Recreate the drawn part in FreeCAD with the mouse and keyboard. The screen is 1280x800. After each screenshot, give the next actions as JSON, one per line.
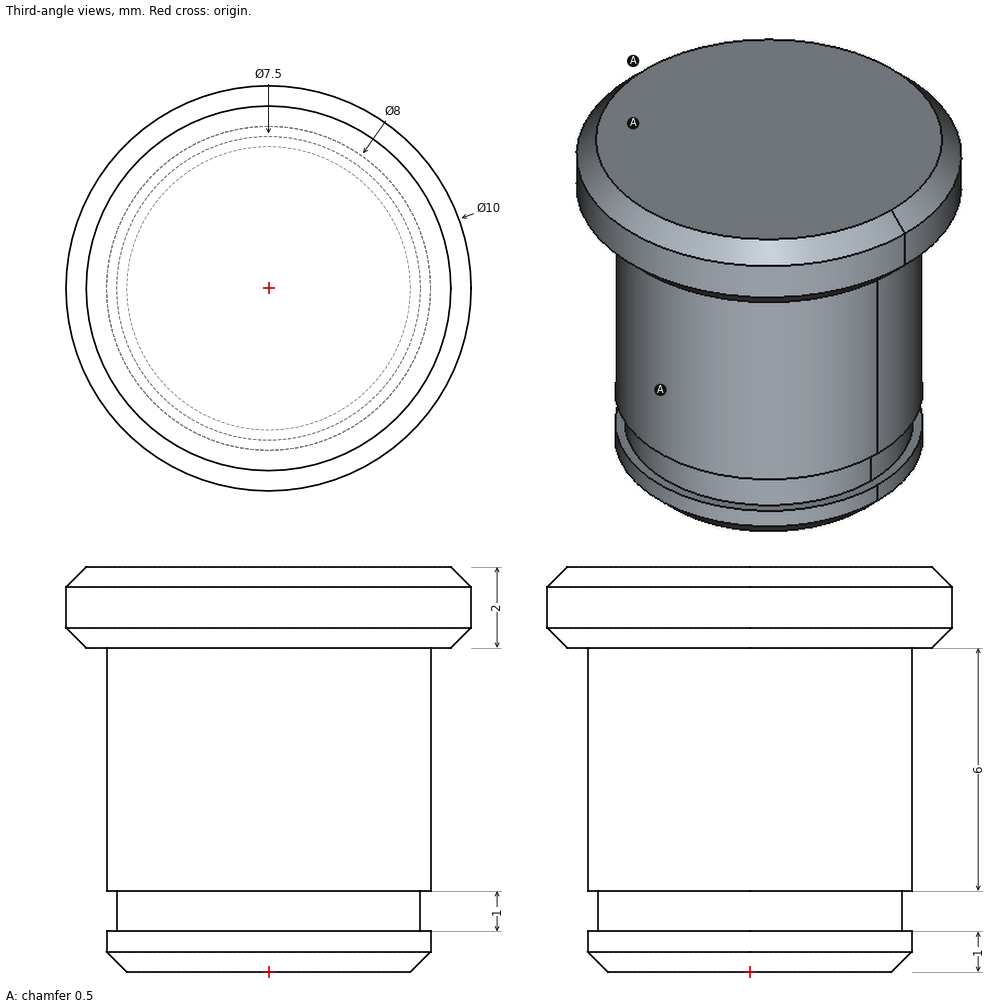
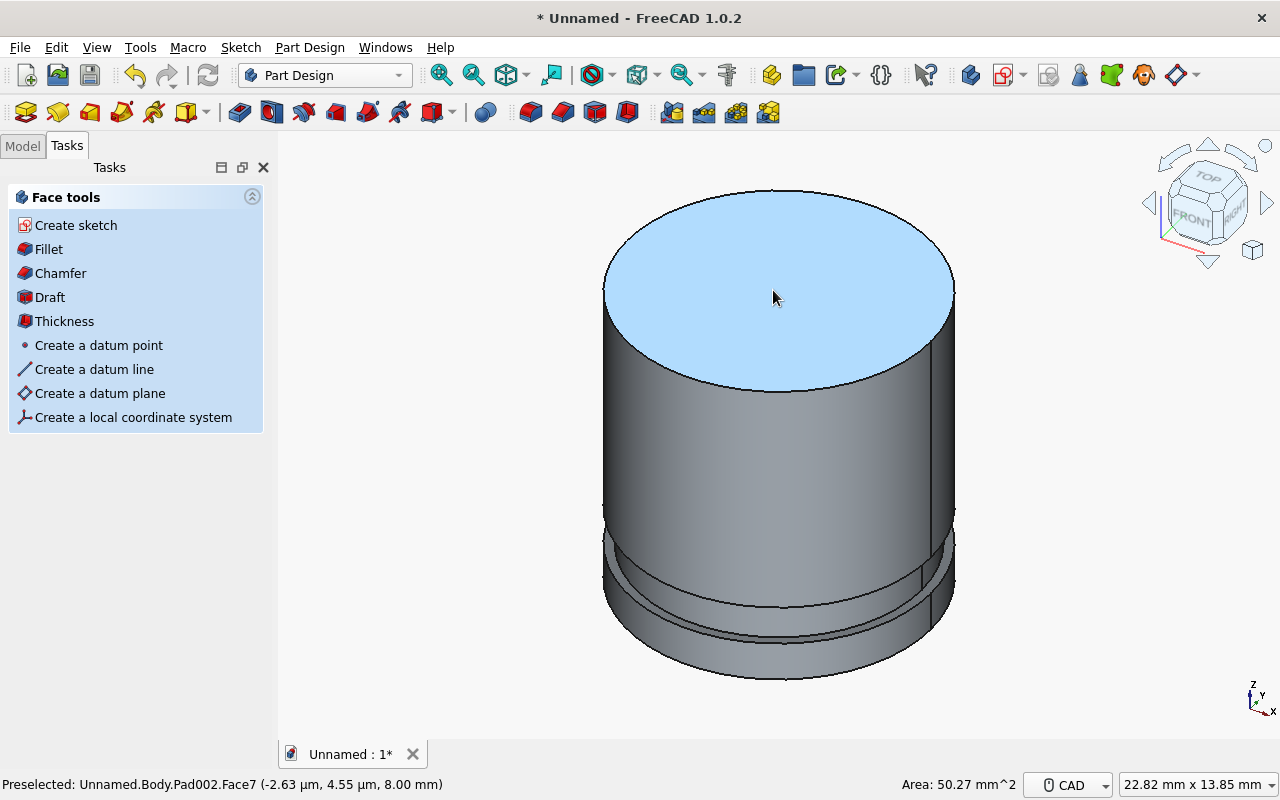
{"action": "left_click", "coordinate": [1004, 76]}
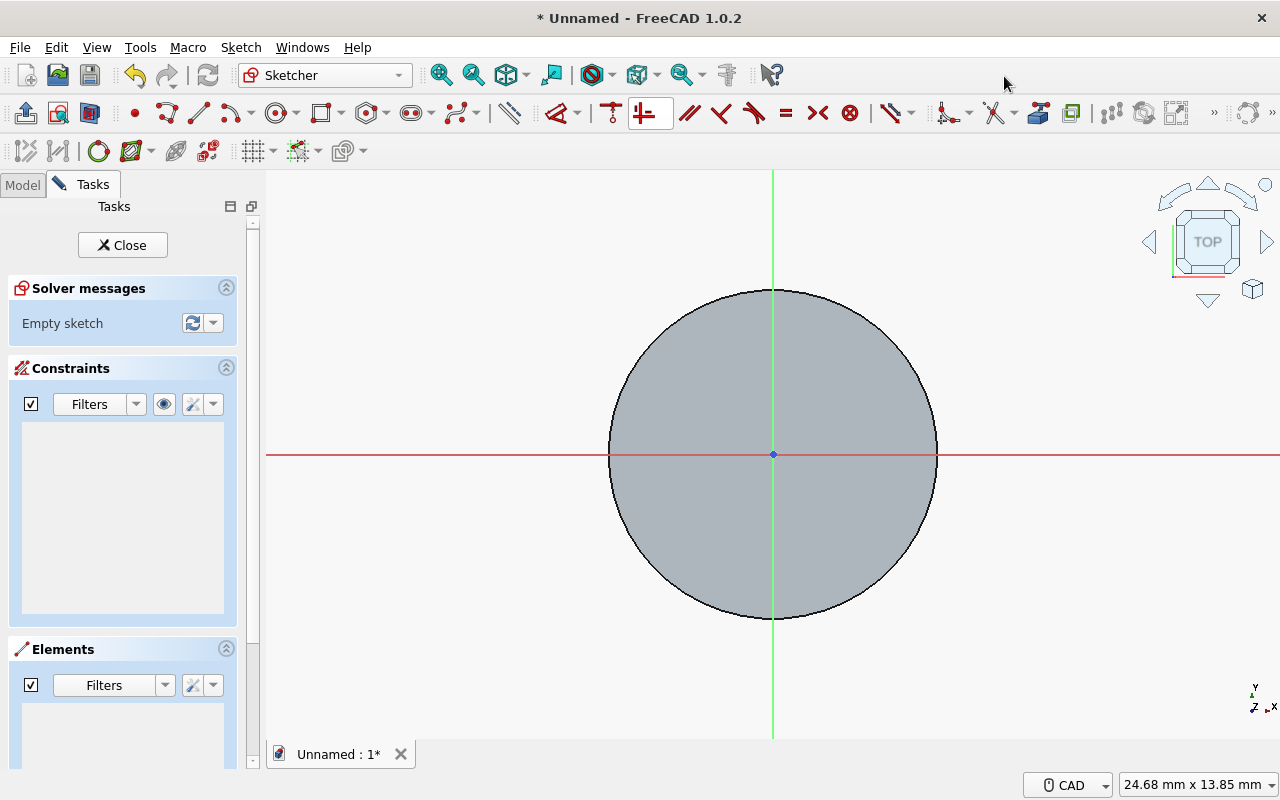
{"action": "key", "text": "g c"}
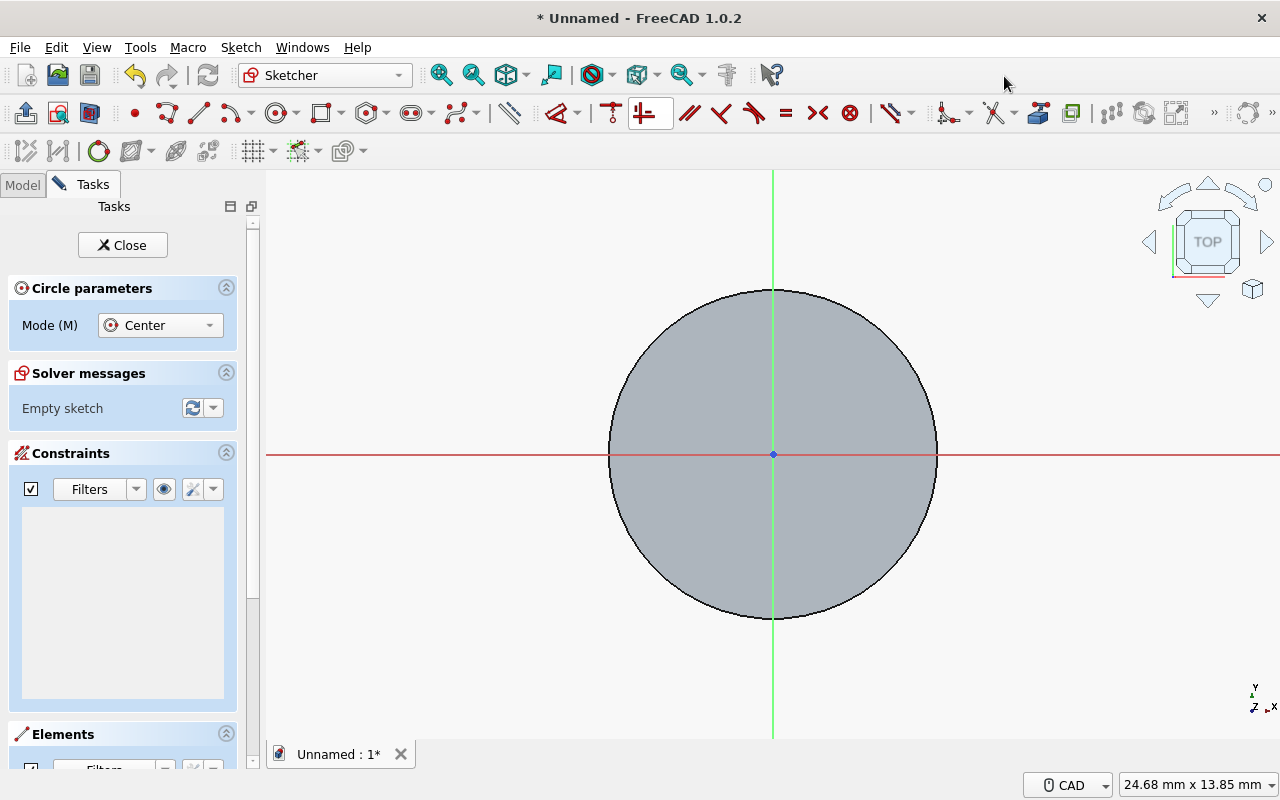
{"action": "left_click", "coordinate": [773, 454]}
{"action": "left_click", "coordinate": [918, 309]}
{"action": "key", "text": "Escape"}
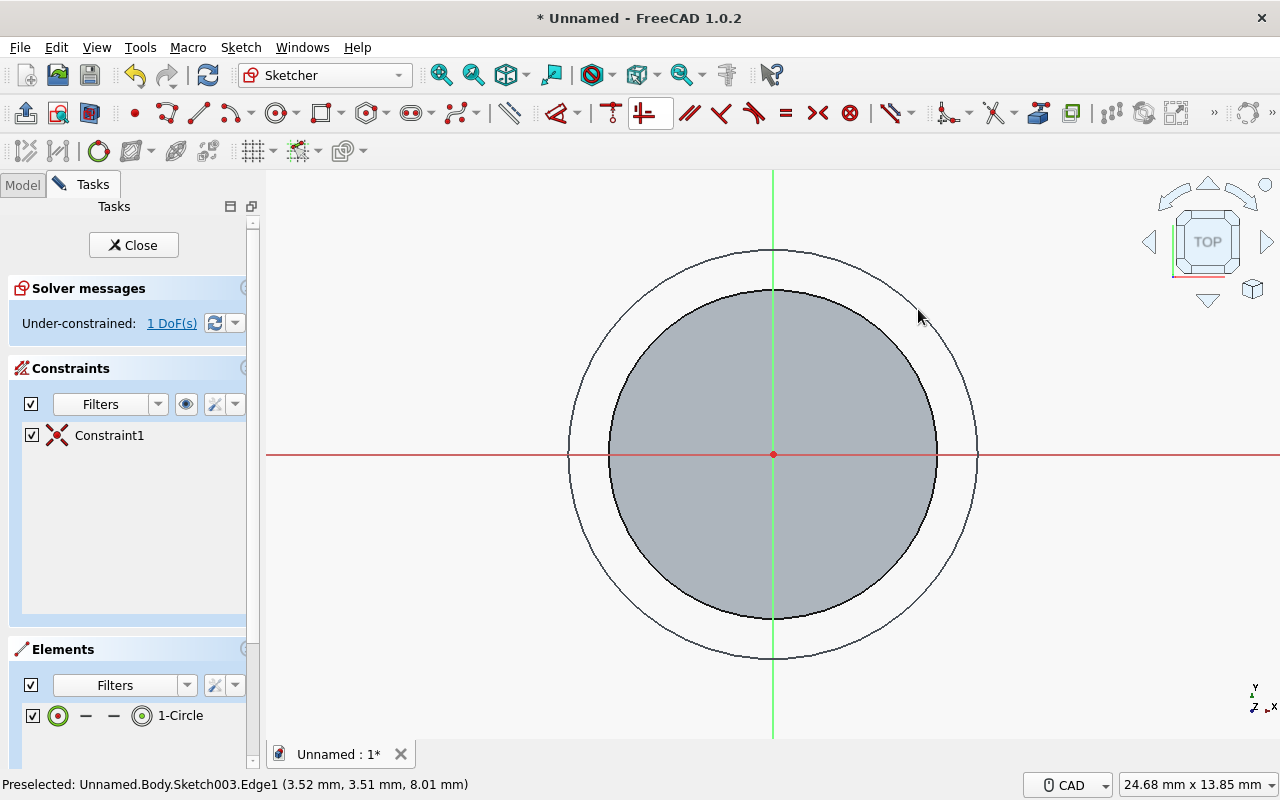
{"action": "key", "text": "d"}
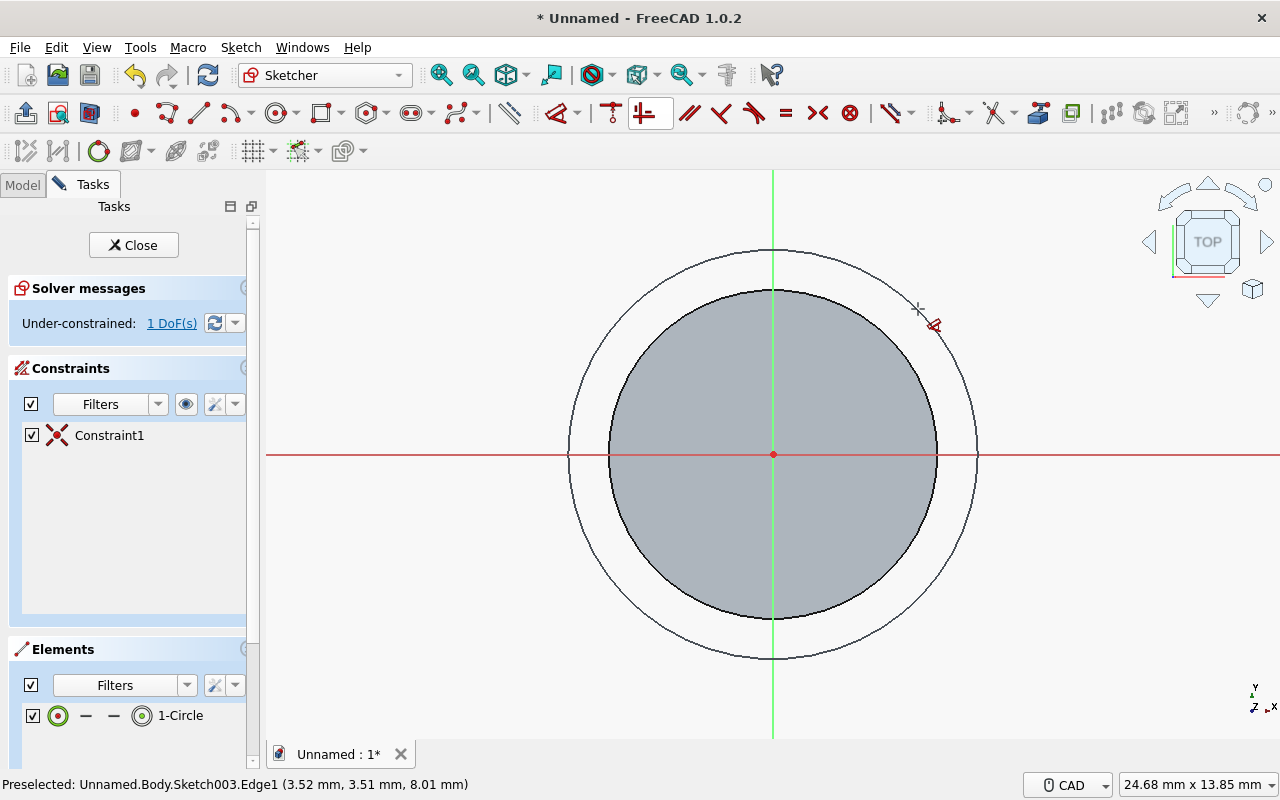
{"action": "left_click", "coordinate": [917, 309]}
{"action": "left_click", "coordinate": [940, 286]}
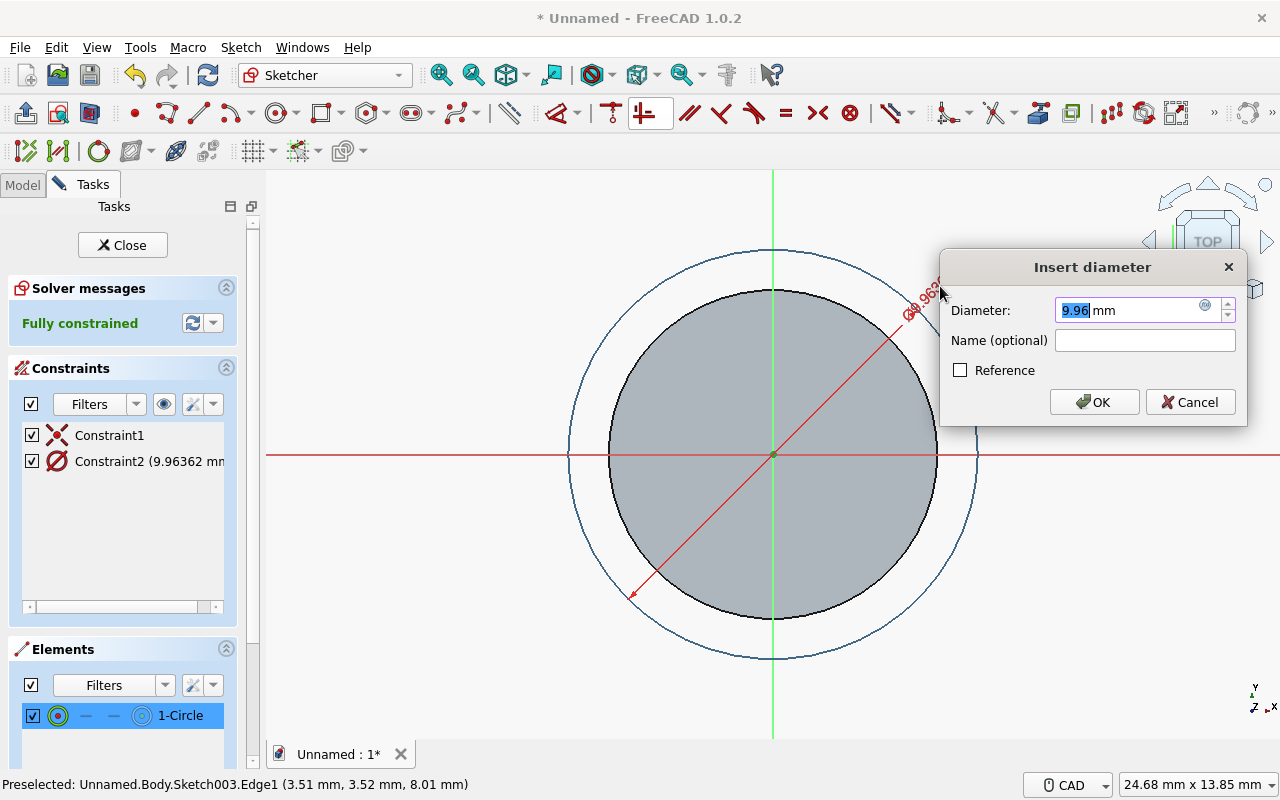
{"action": "type", "text": "10"}
{"action": "key", "text": "Return"}
{"action": "key", "text": "Escape"}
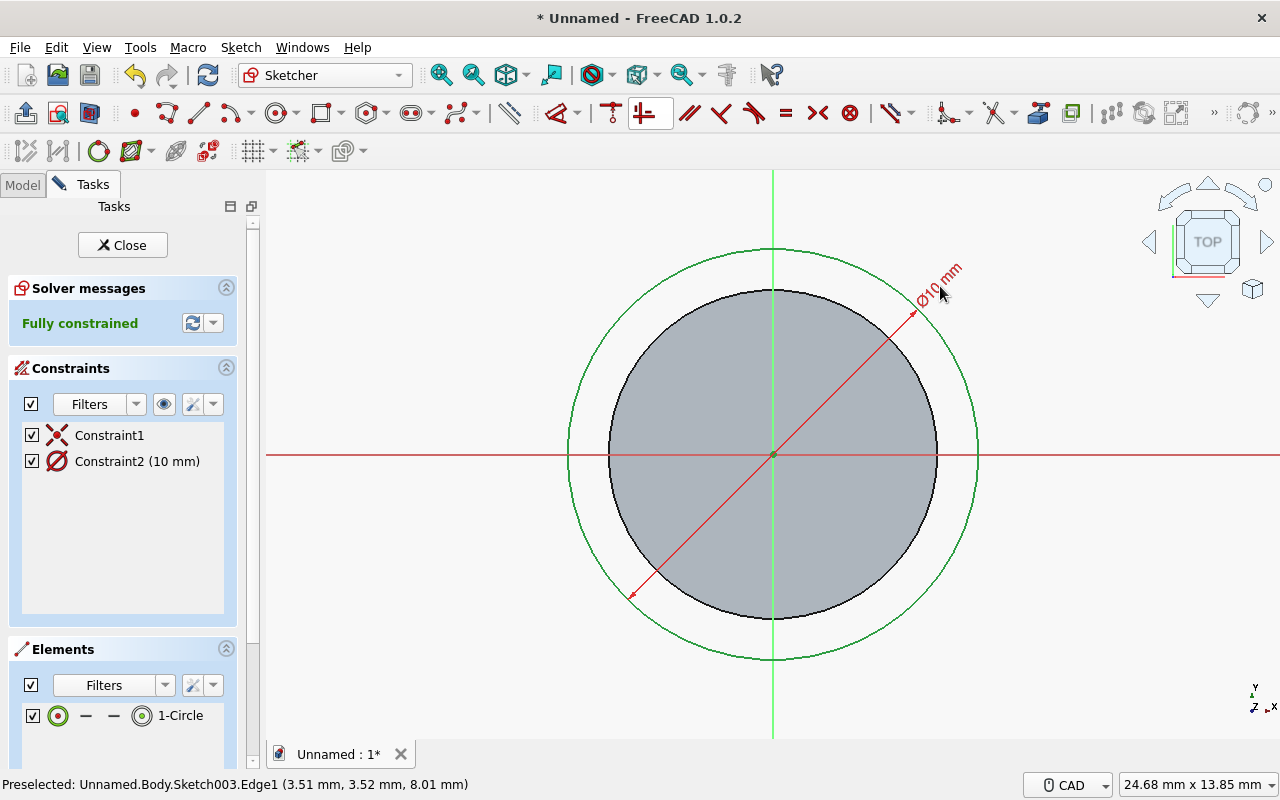
{"action": "left_click", "coordinate": [123, 245]}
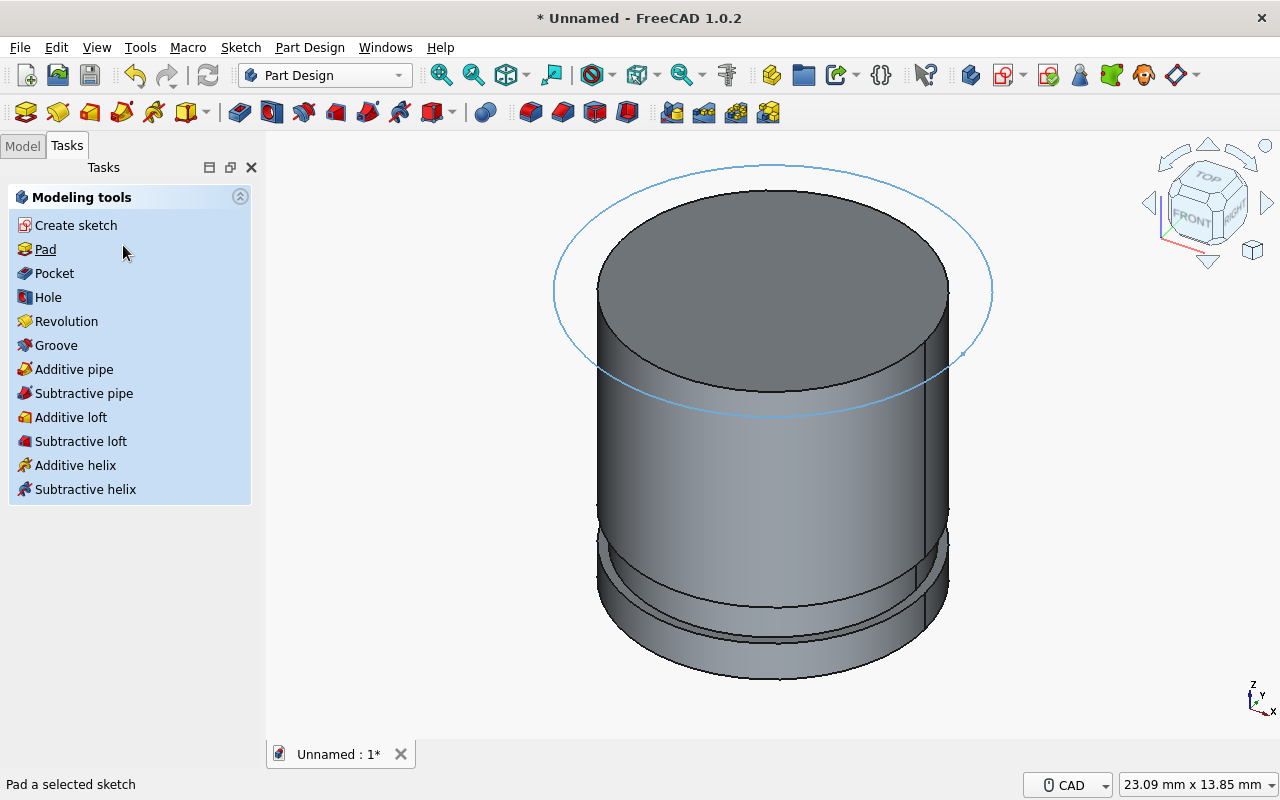
{"action": "left_click", "coordinate": [26, 112]}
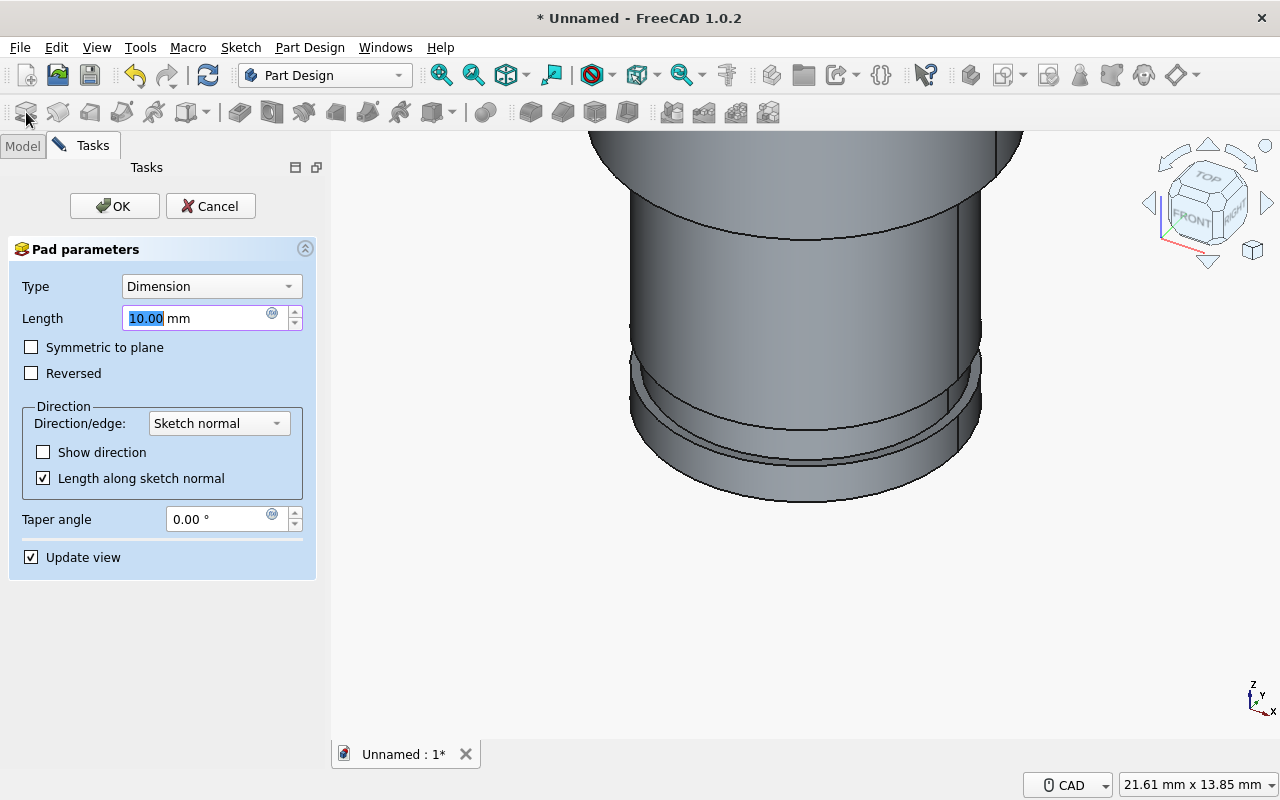
{"action": "type", "text": "2"}
{"action": "key", "text": "Tab"}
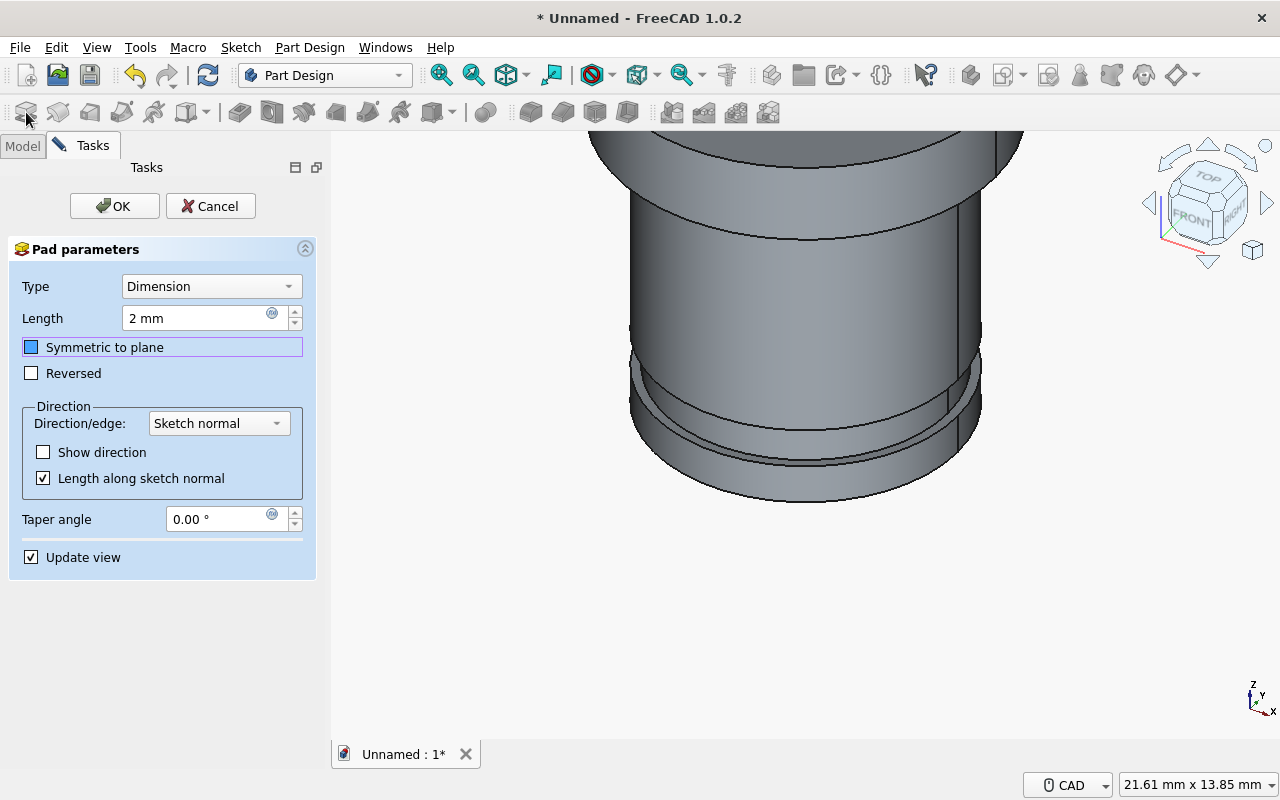
{"action": "left_click", "coordinate": [115, 206]}